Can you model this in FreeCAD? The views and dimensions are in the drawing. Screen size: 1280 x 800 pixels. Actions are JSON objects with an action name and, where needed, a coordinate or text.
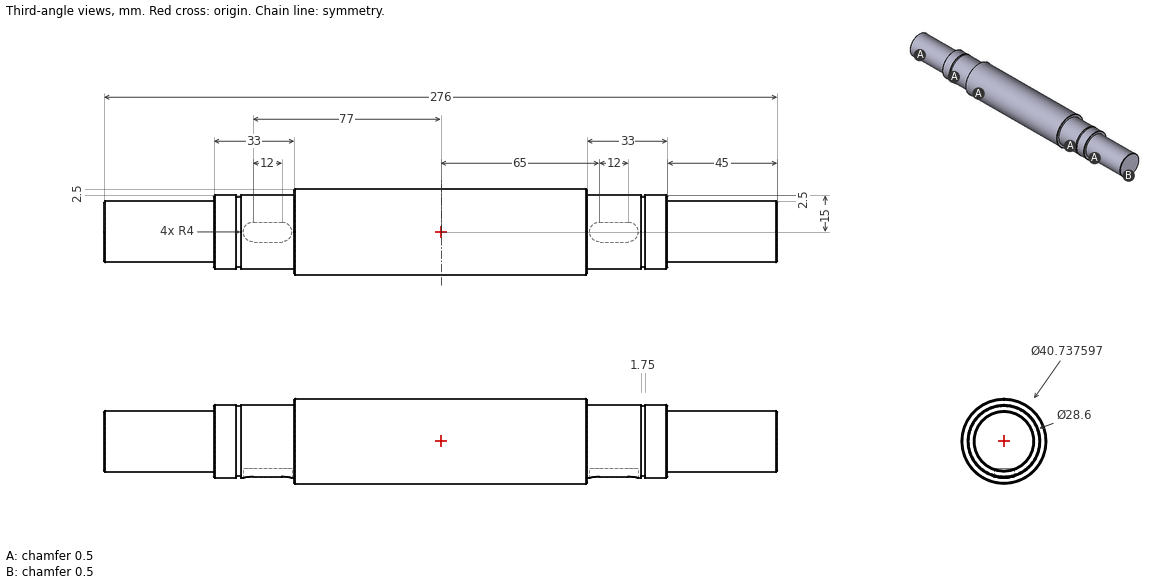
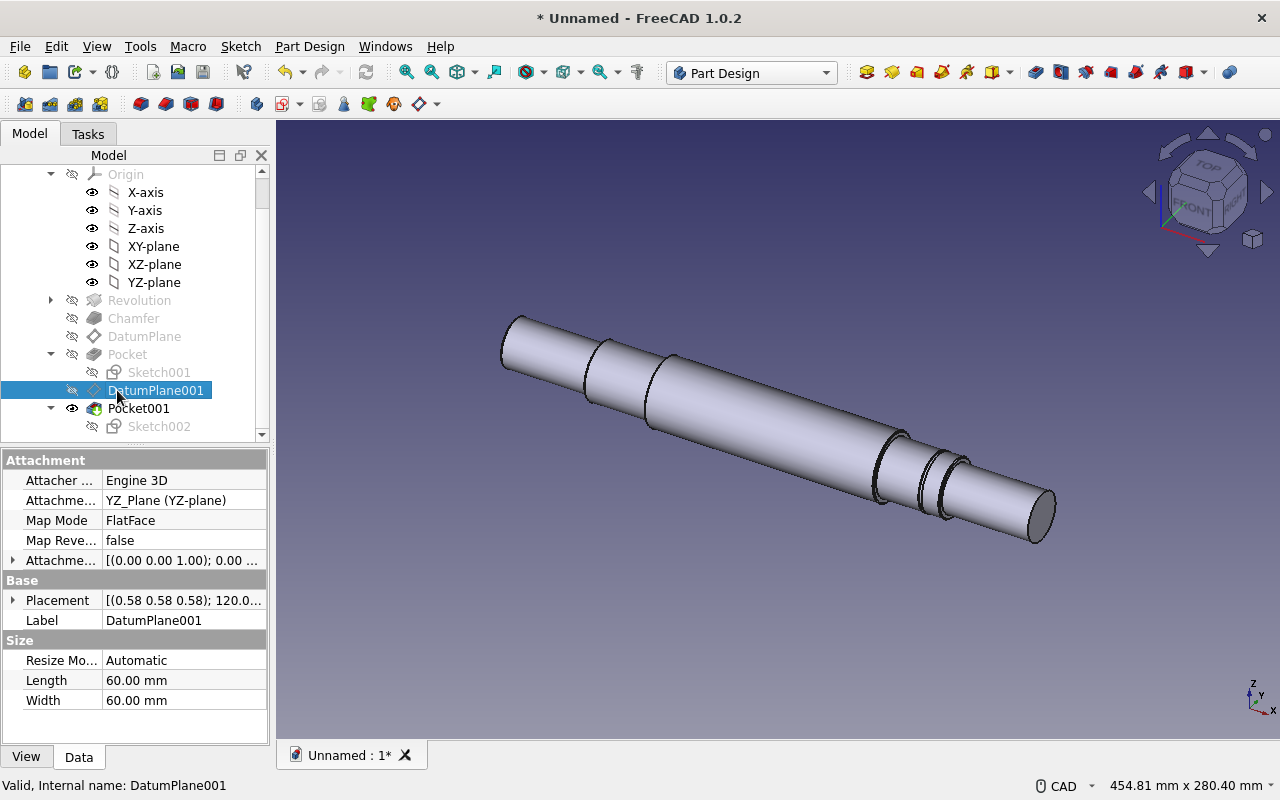
{"action": "left_click", "coordinate": [117, 408]}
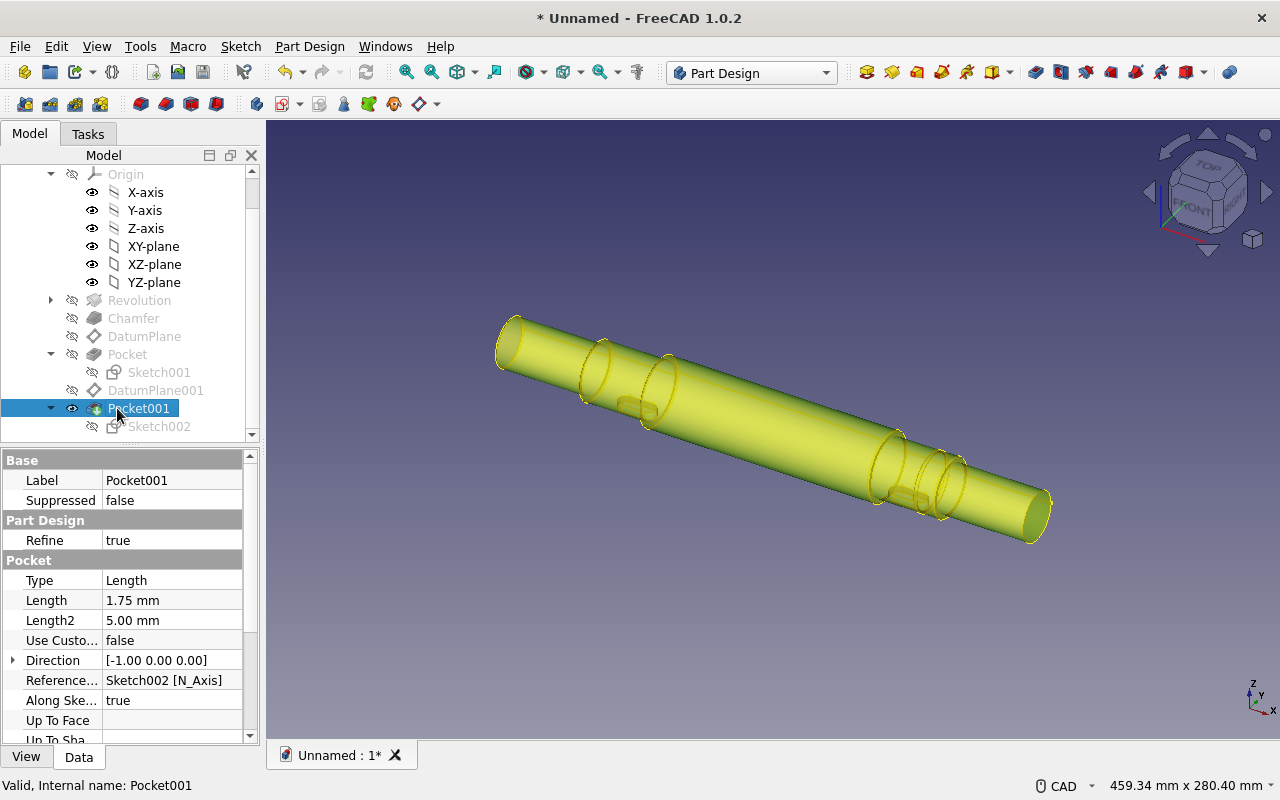
{"action": "left_click", "coordinate": [25, 104]}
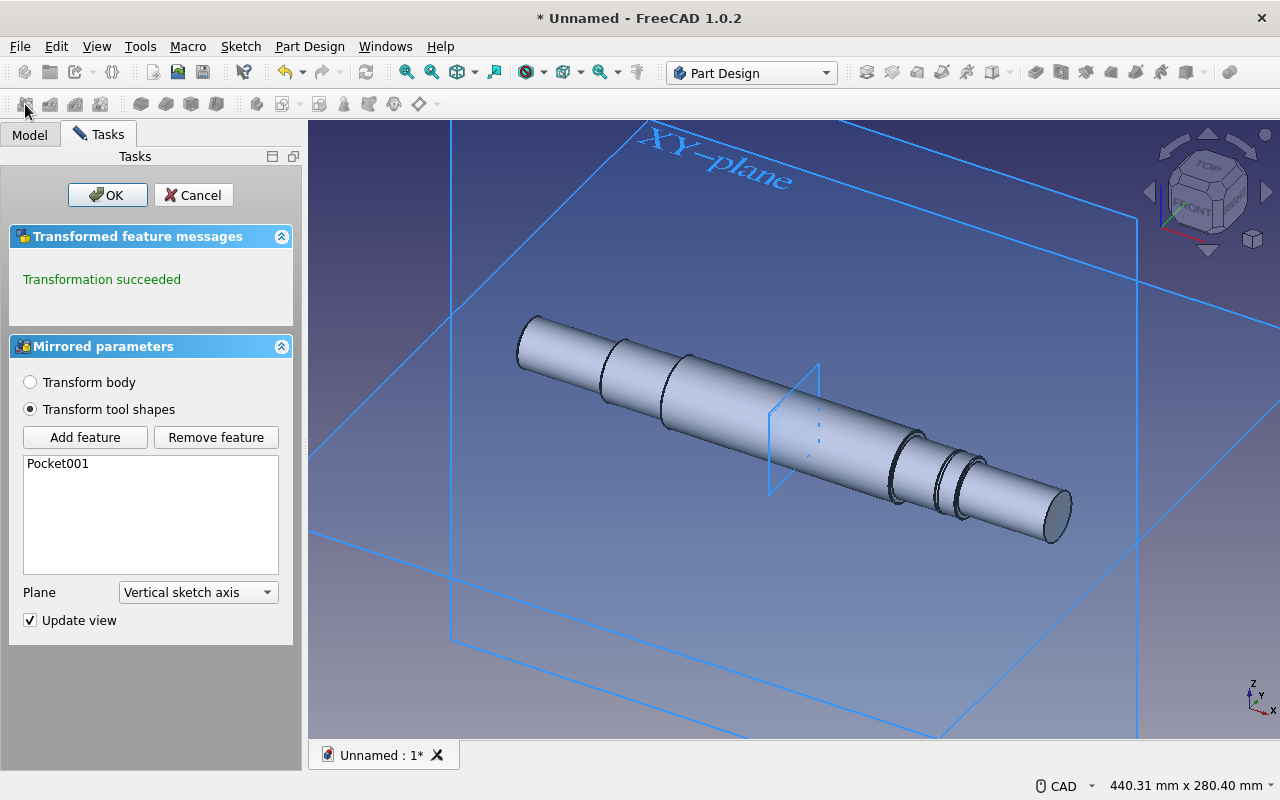
{"action": "left_click", "coordinate": [199, 592]}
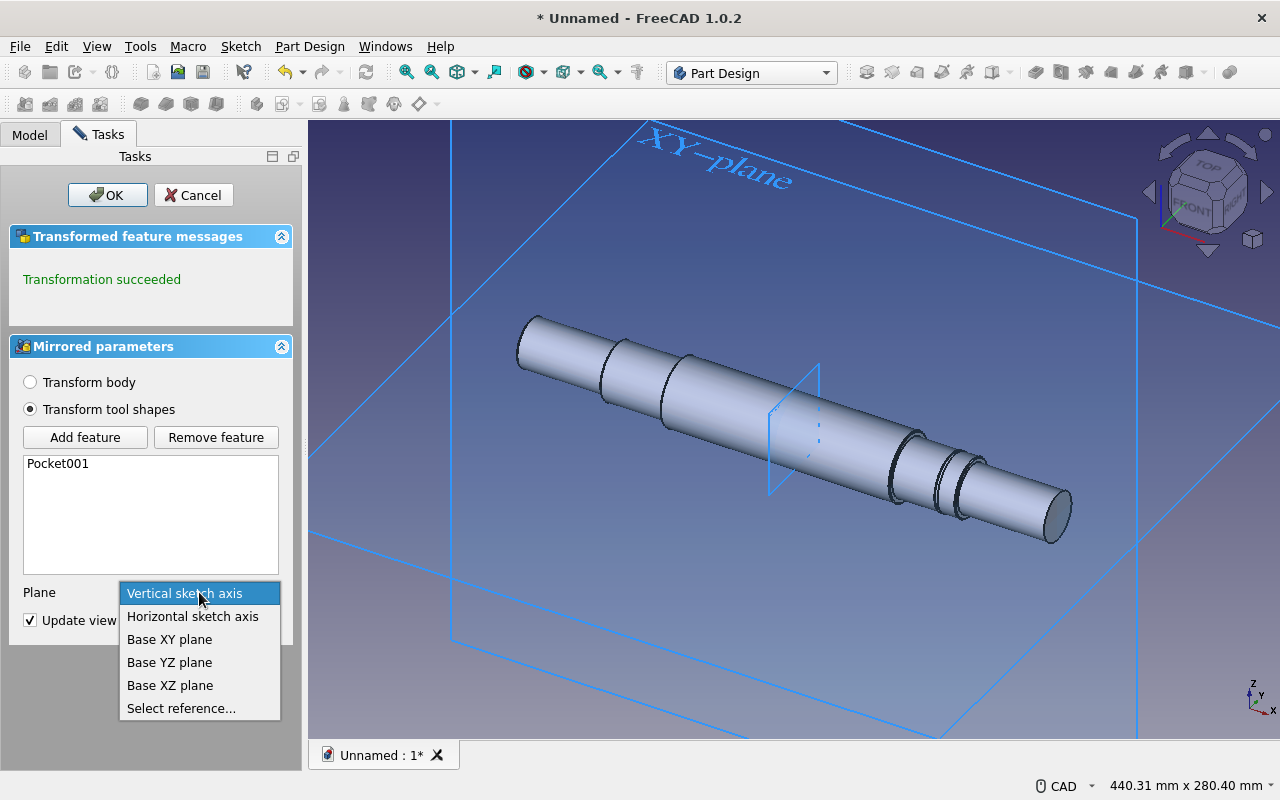
{"action": "left_click", "coordinate": [198, 662]}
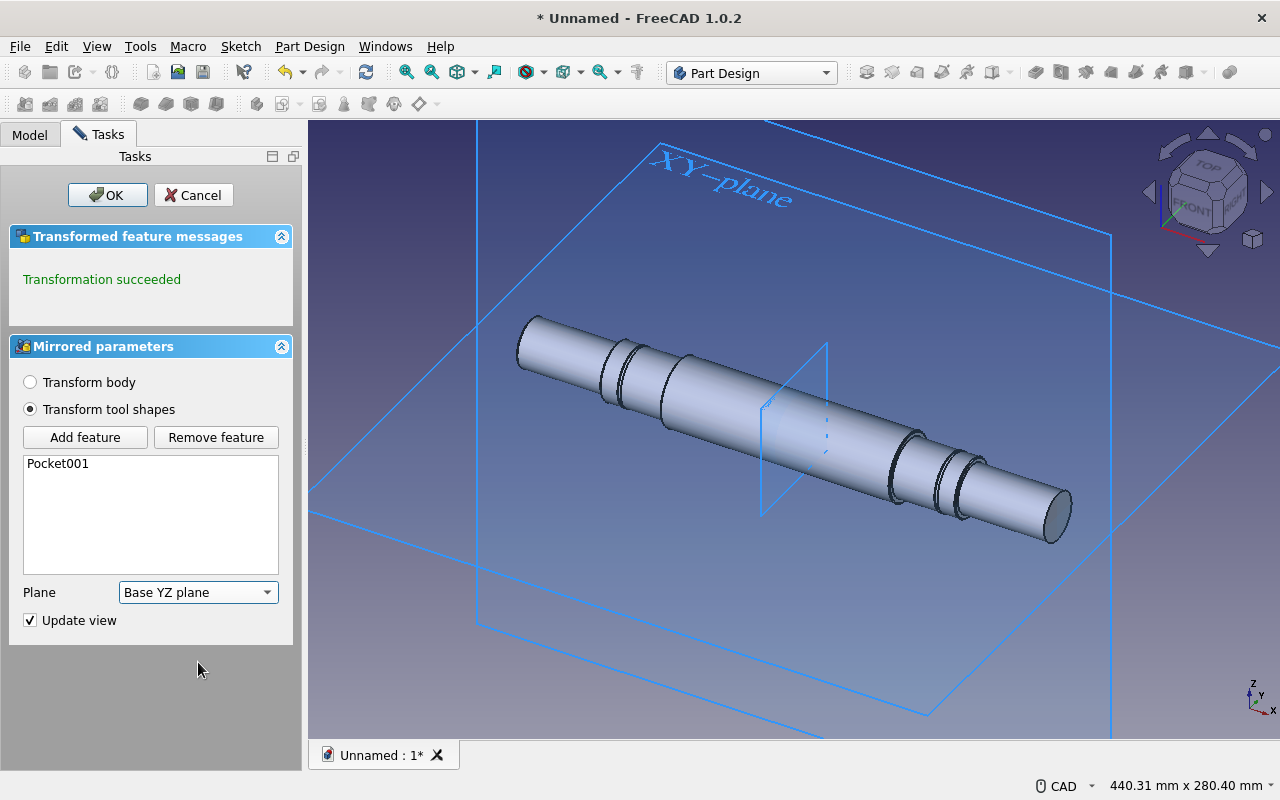
{"action": "left_click", "coordinate": [108, 195]}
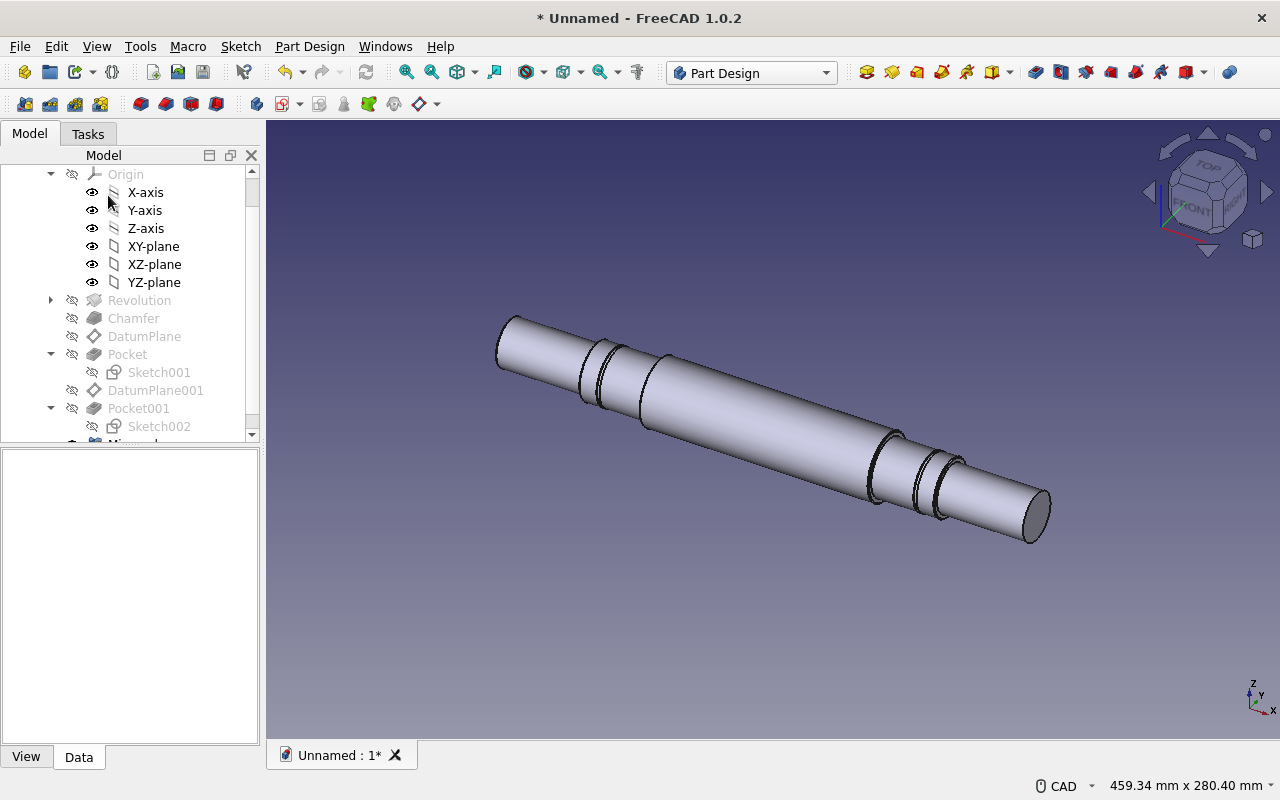
{"action": "left_click", "coordinate": [1023, 530]}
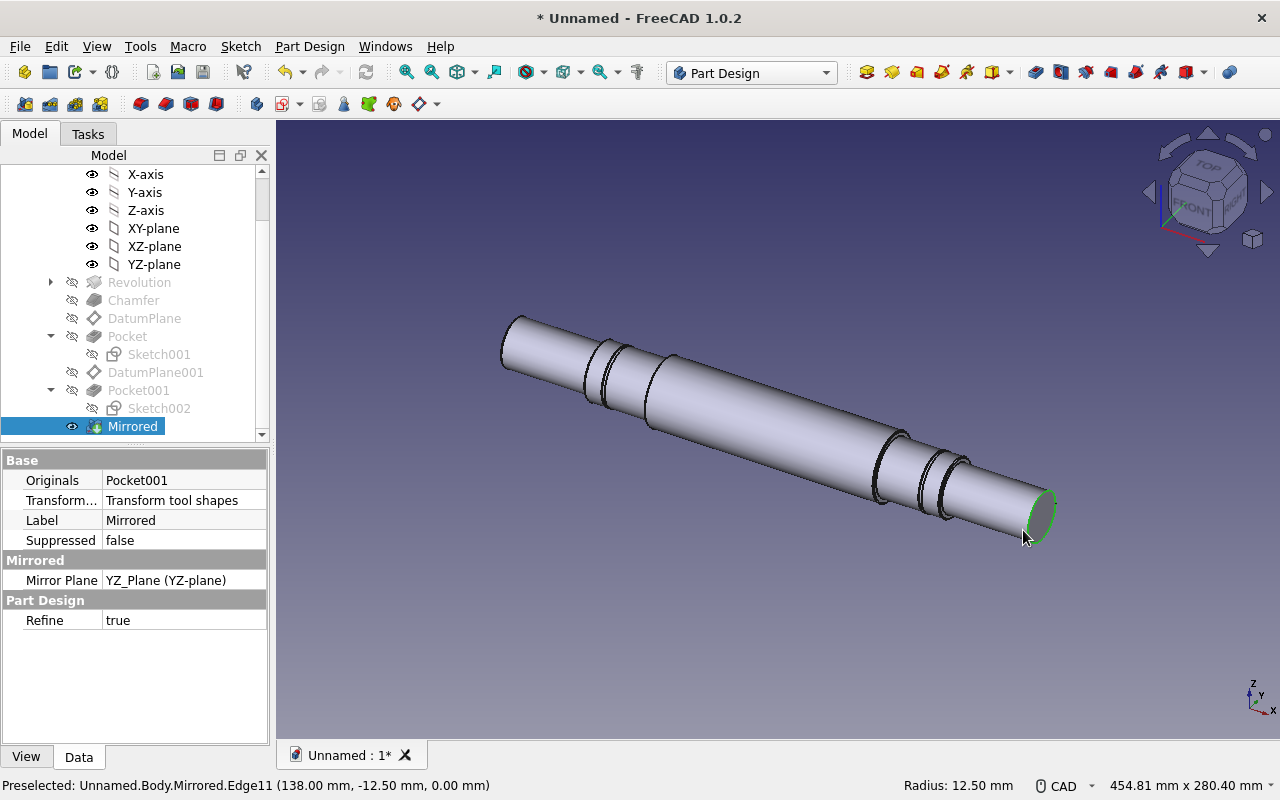
{"action": "left_click", "coordinate": [166, 104]}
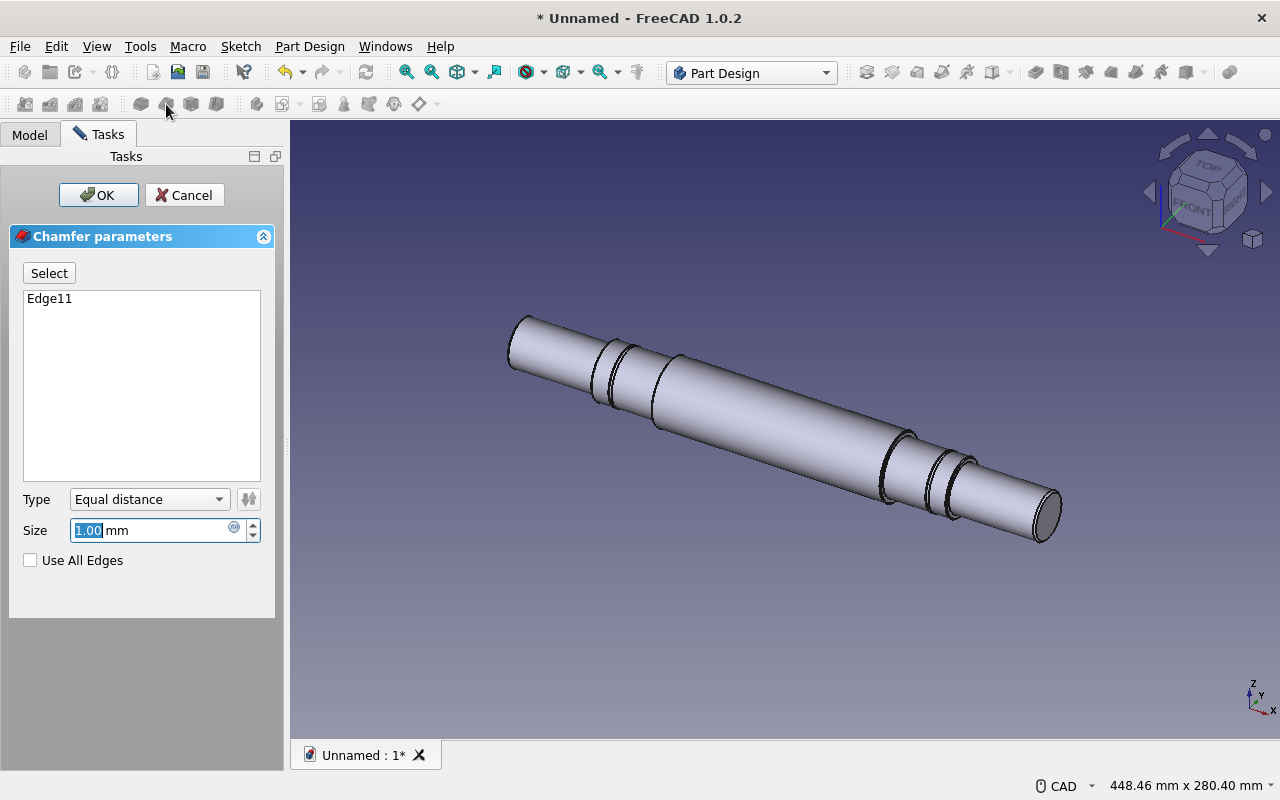
{"action": "type", "text": "0.5"}
{"action": "key", "text": "Tab"}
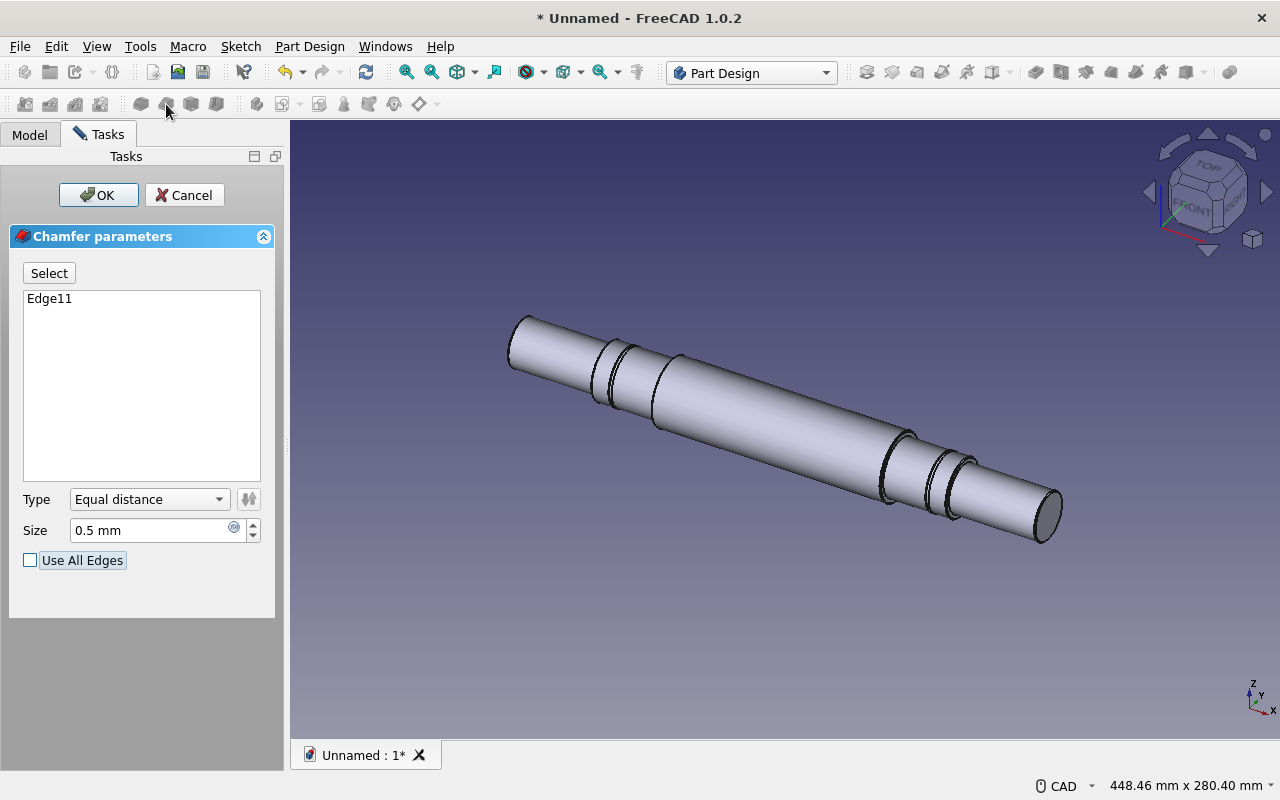
{"action": "left_click", "coordinate": [99, 195]}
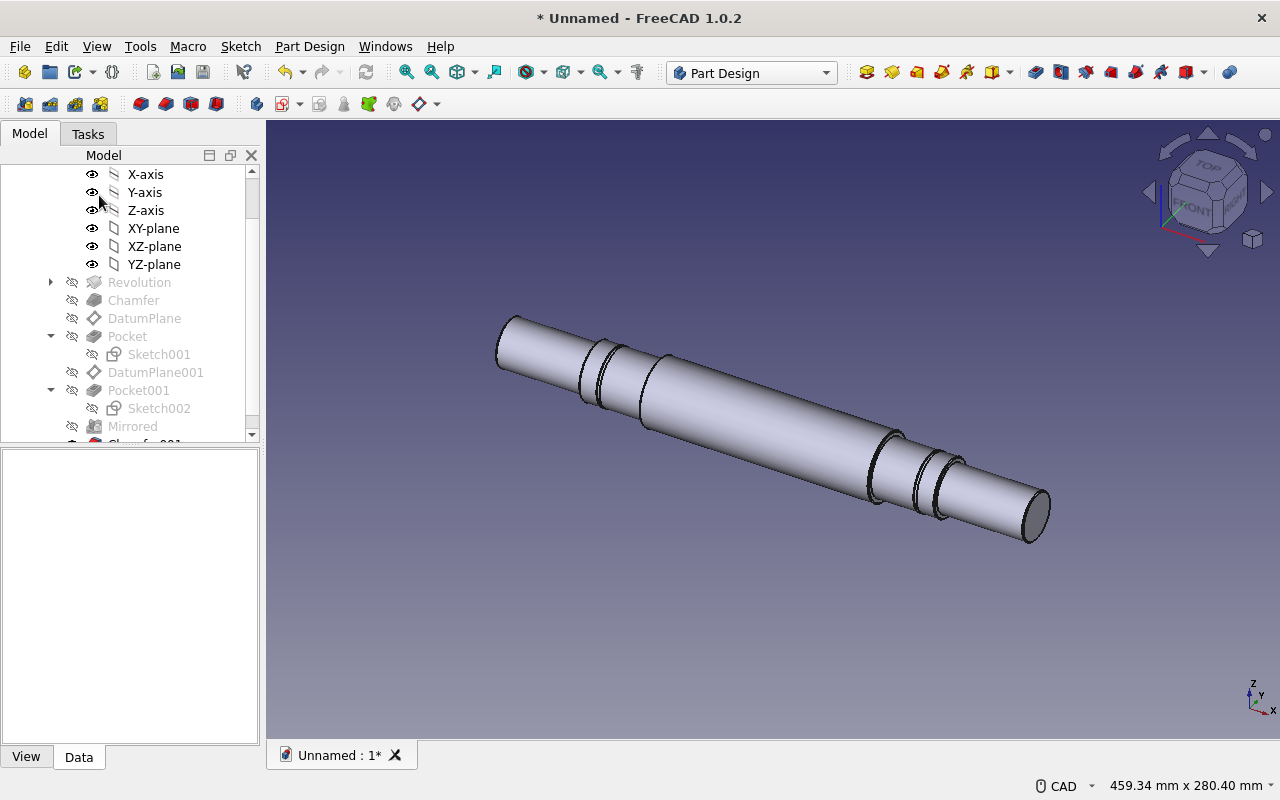
{"action": "key", "text": "0"}